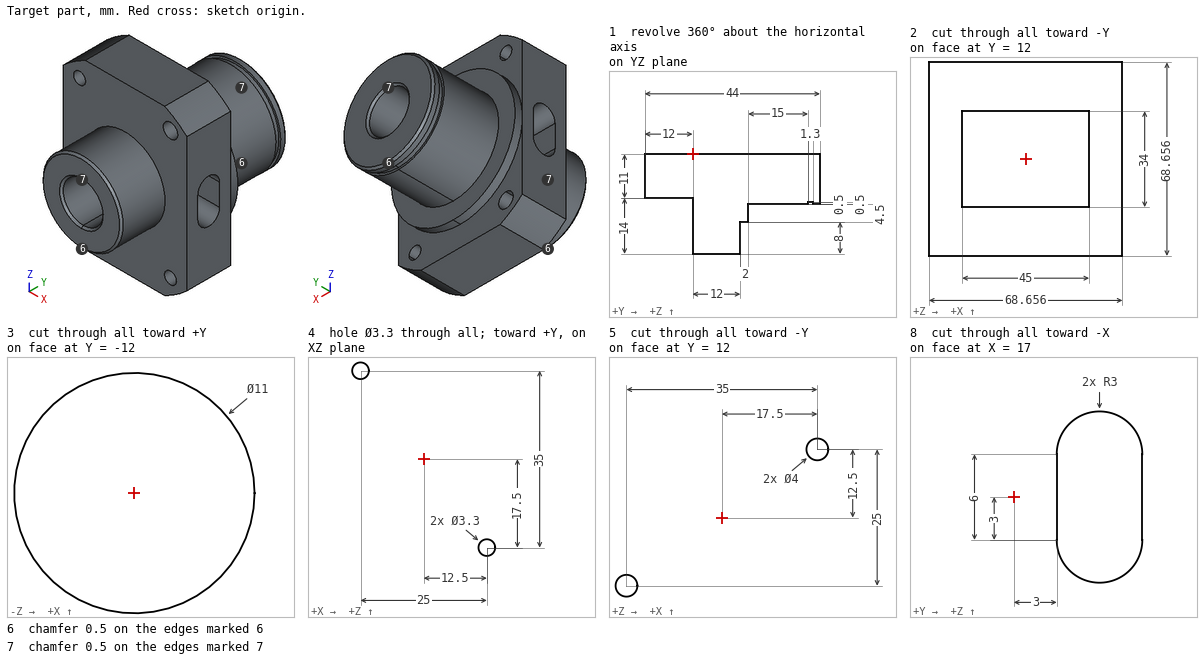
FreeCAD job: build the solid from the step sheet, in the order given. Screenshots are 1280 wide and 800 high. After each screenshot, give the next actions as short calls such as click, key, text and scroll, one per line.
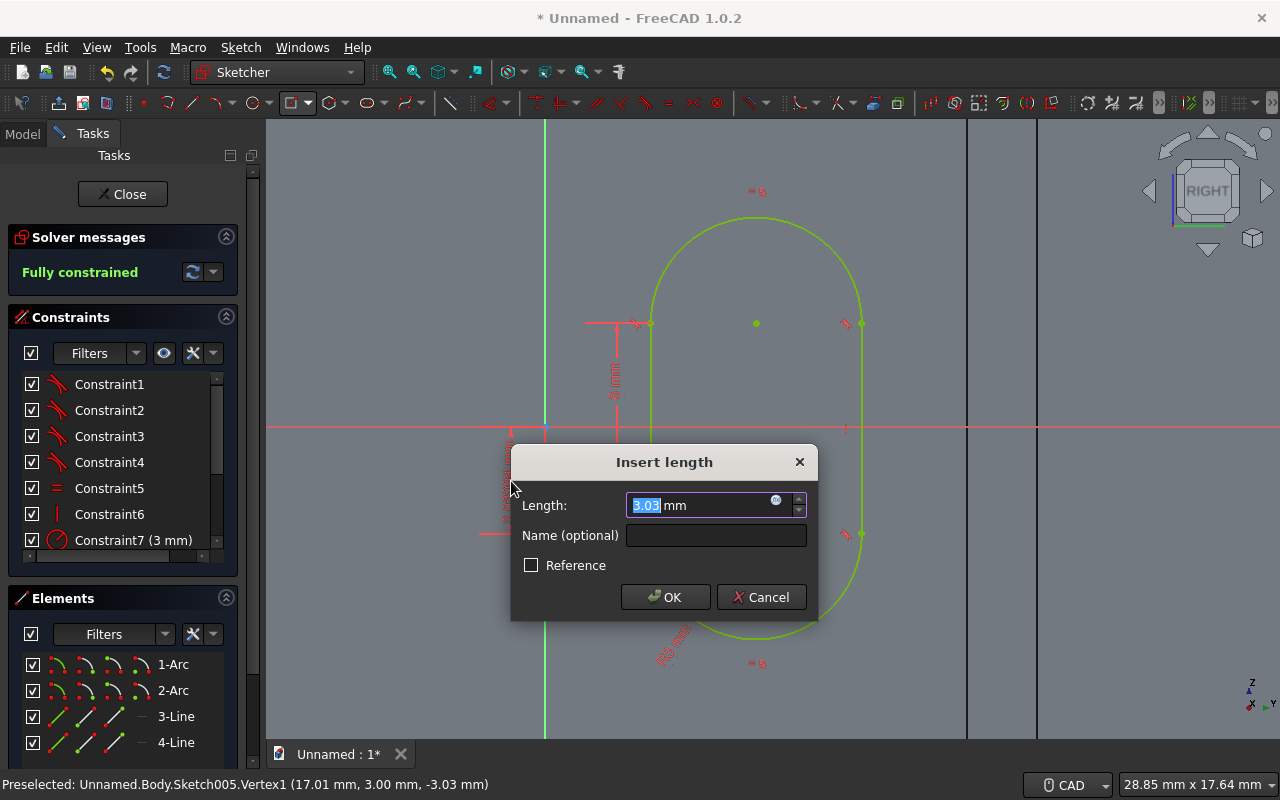
text(3)
key(Return)
key(Escape)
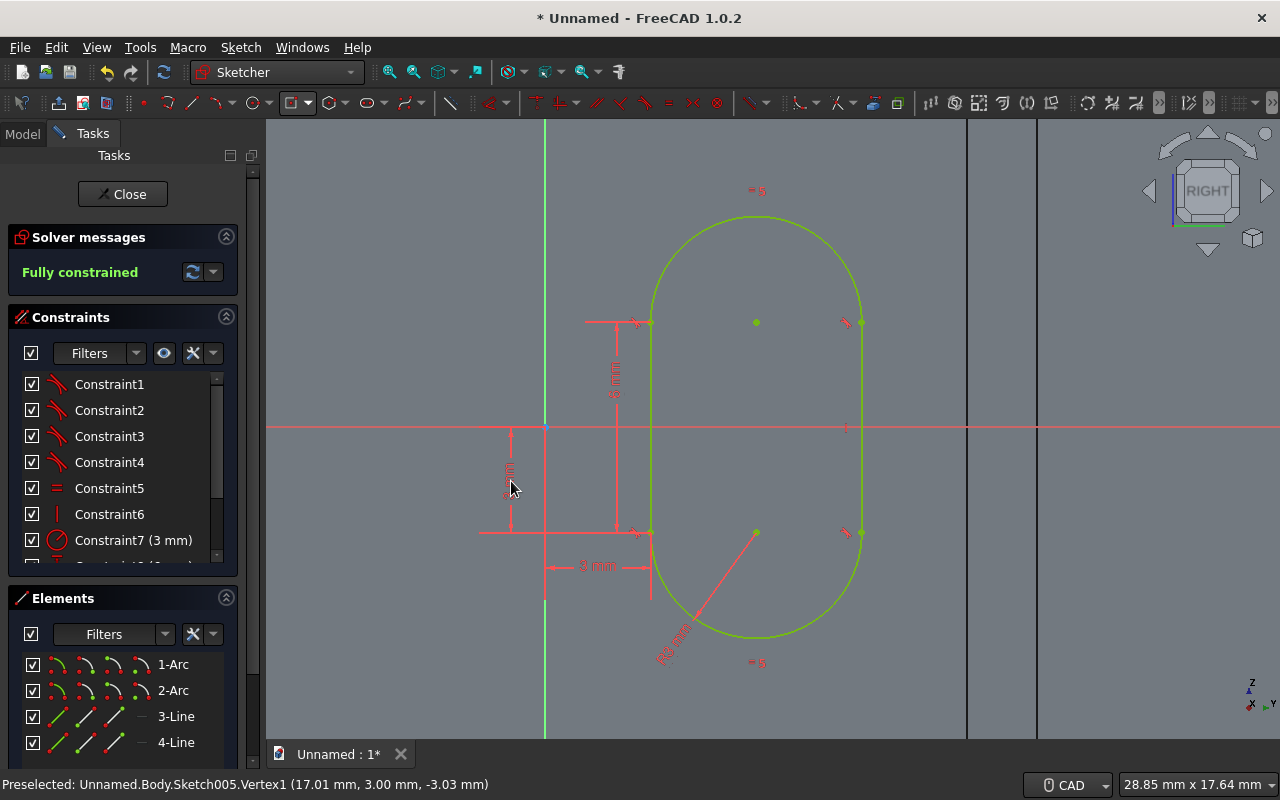
click(123, 194)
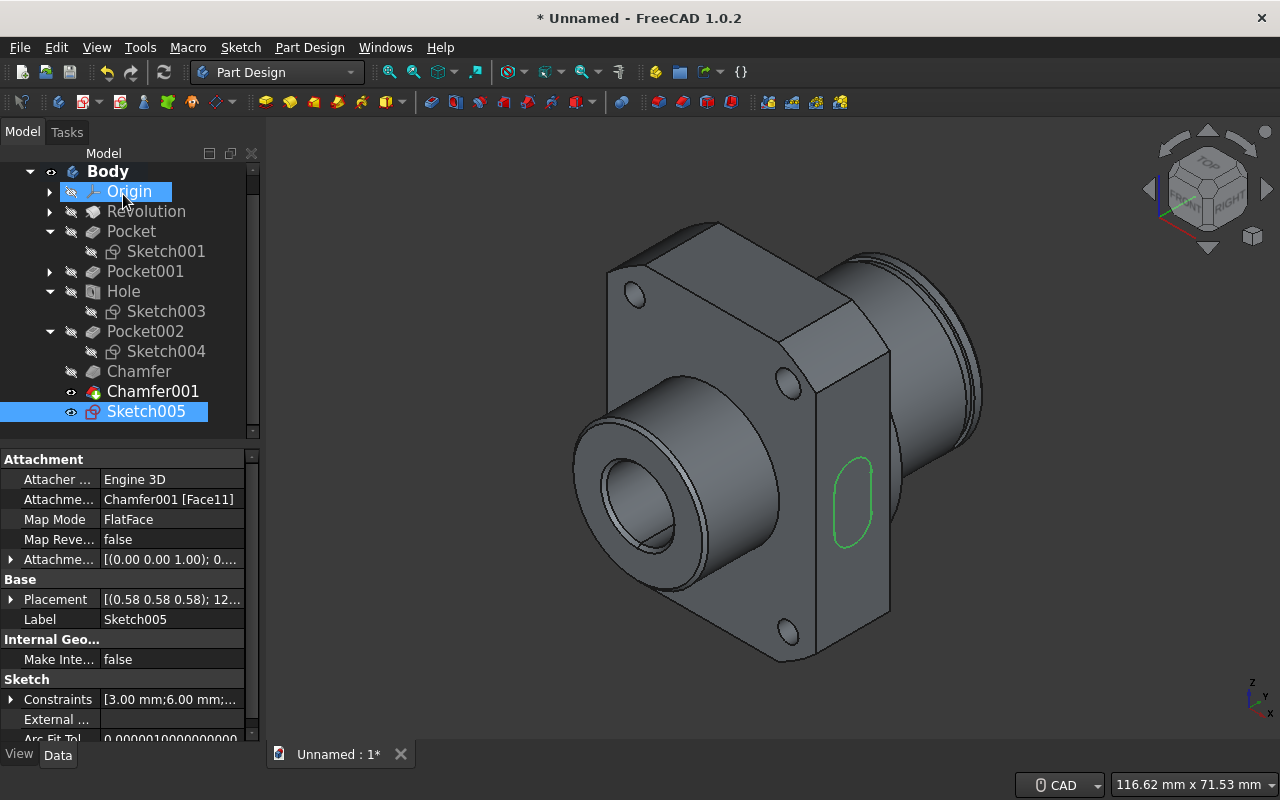
click(432, 102)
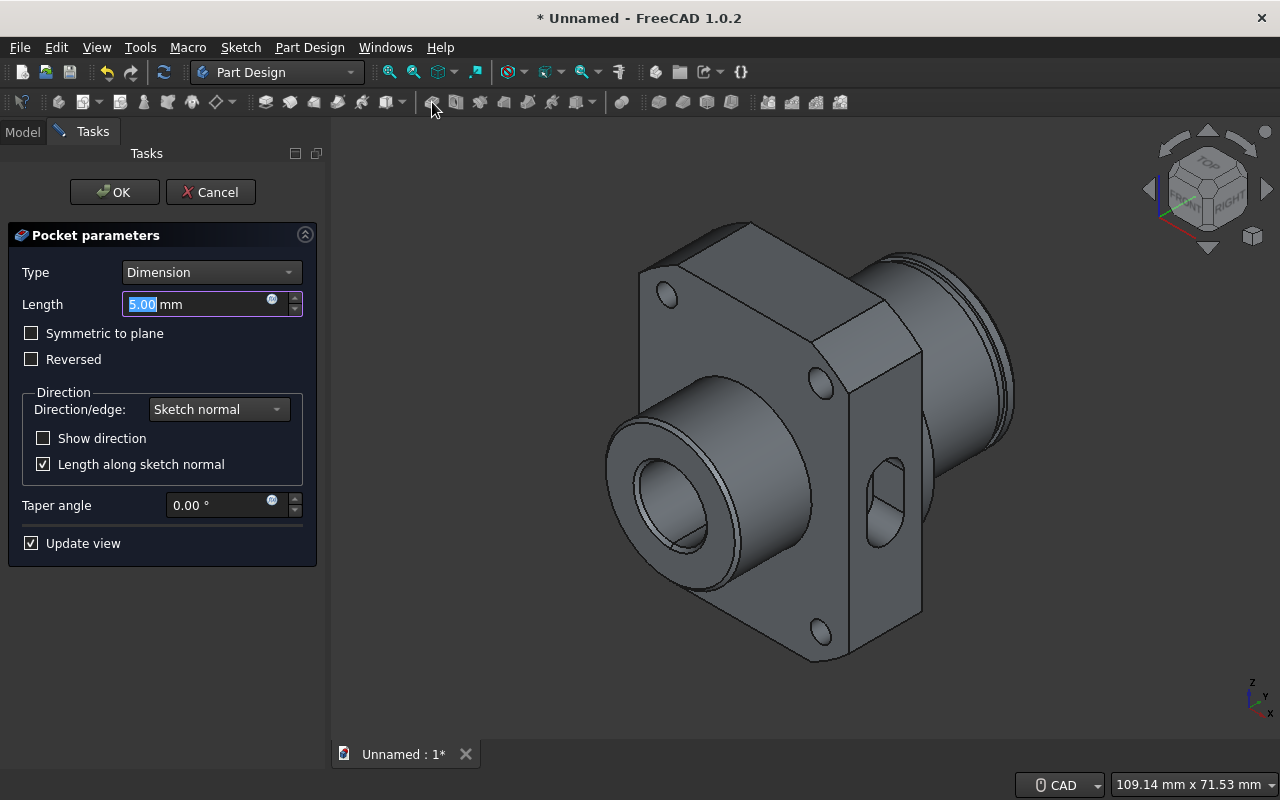
click(212, 272)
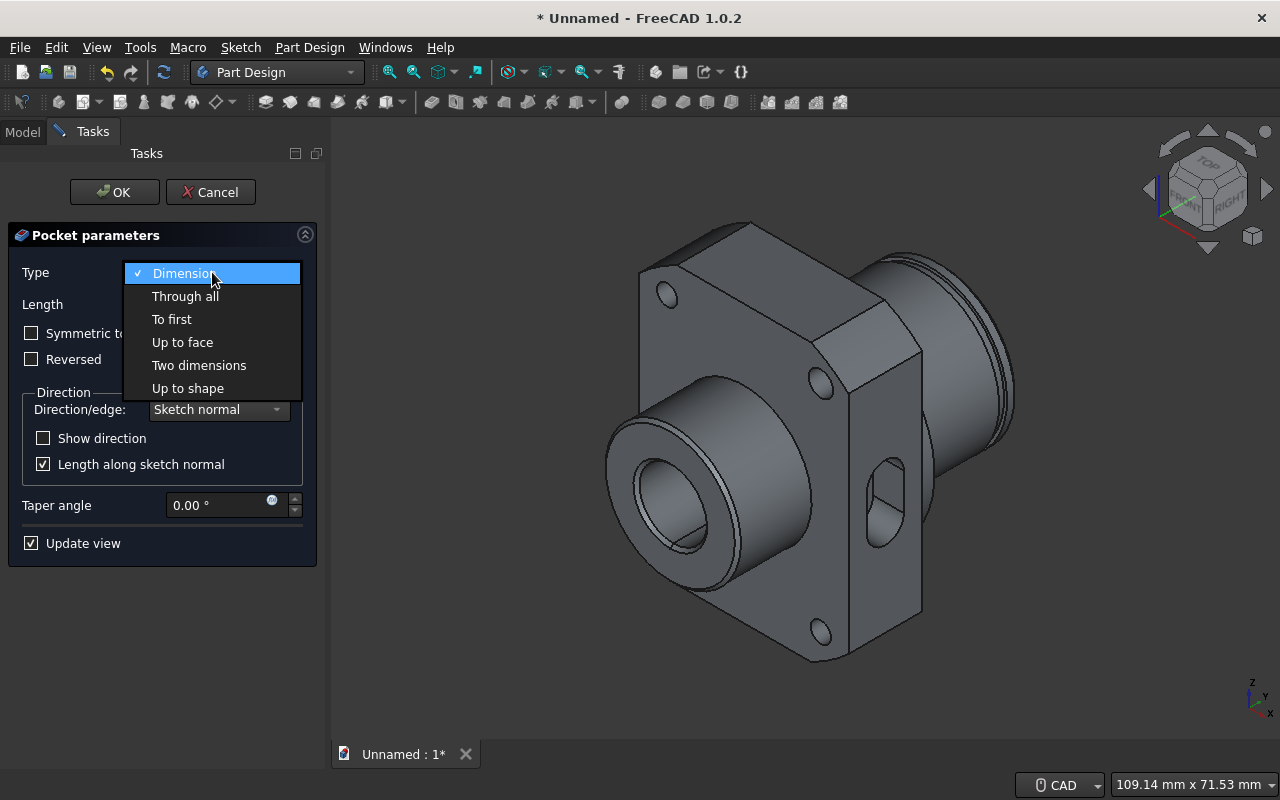
click(212, 296)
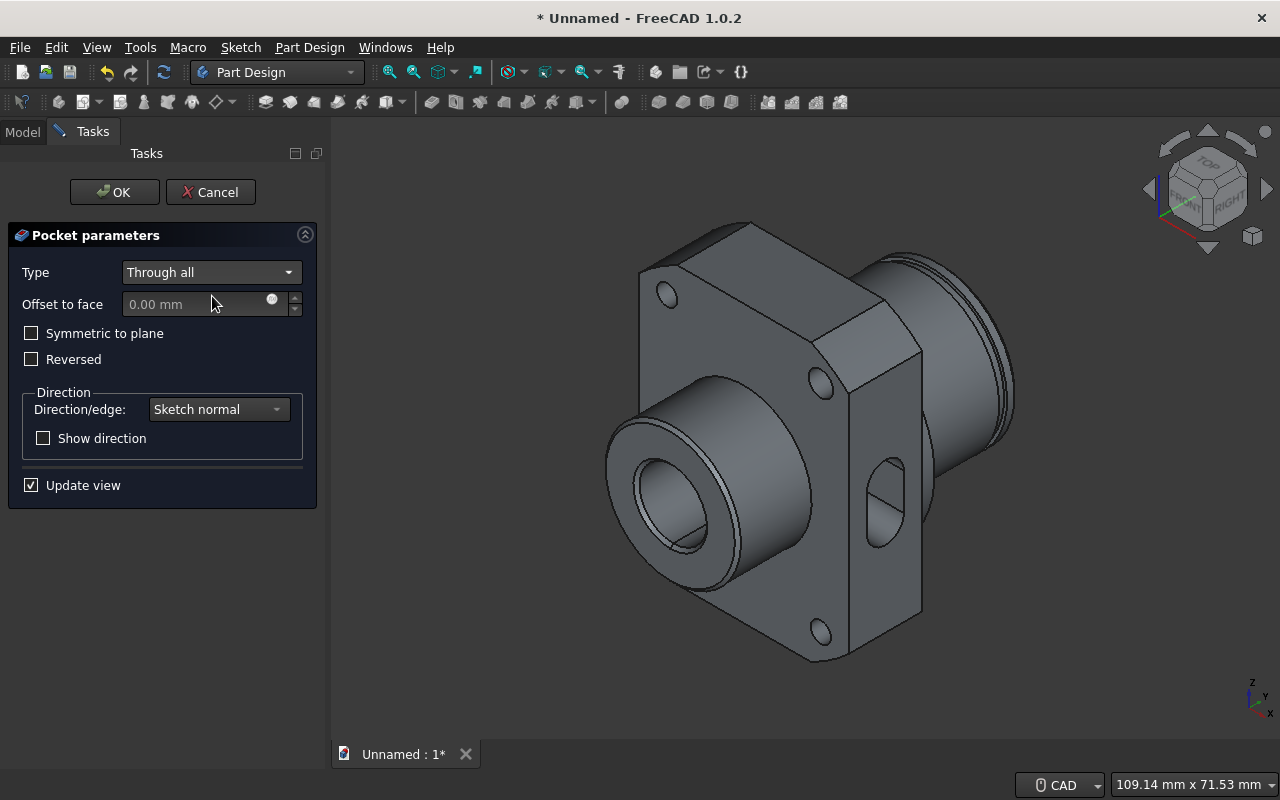
click(115, 192)